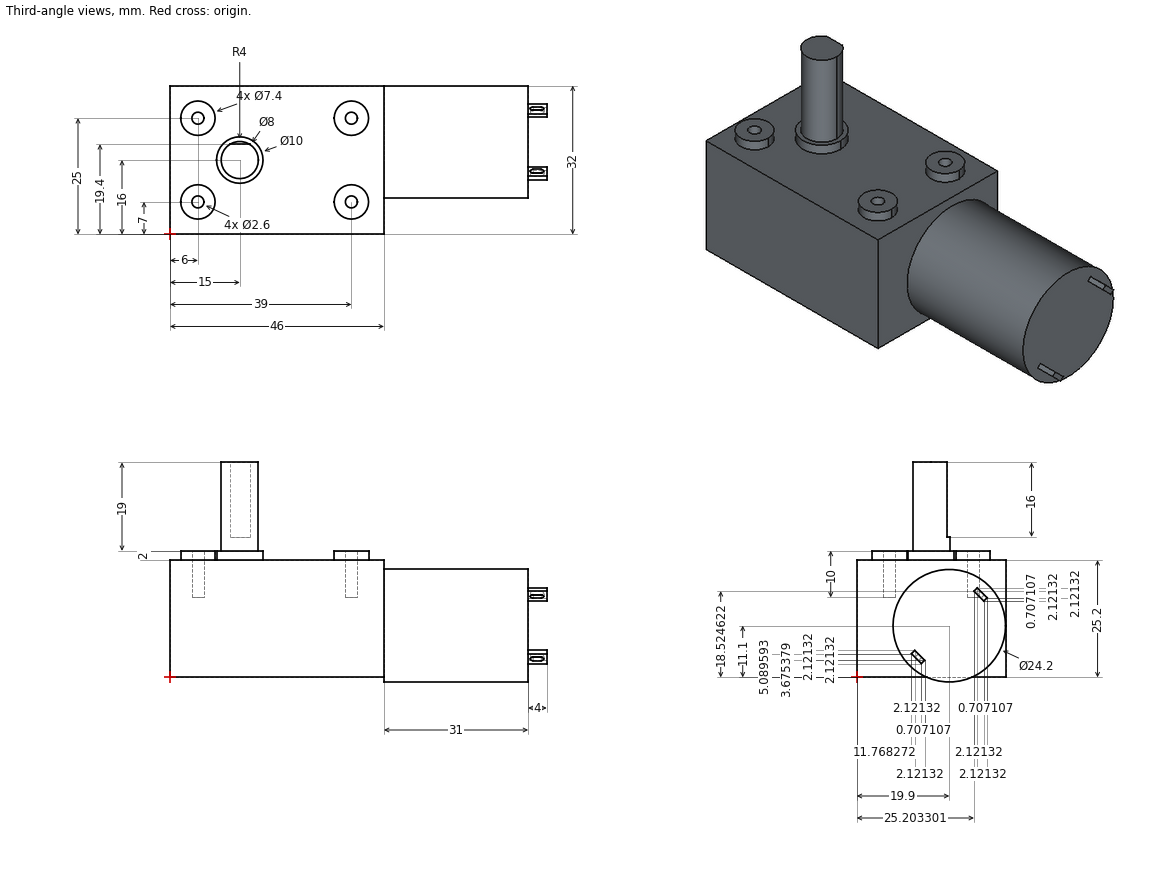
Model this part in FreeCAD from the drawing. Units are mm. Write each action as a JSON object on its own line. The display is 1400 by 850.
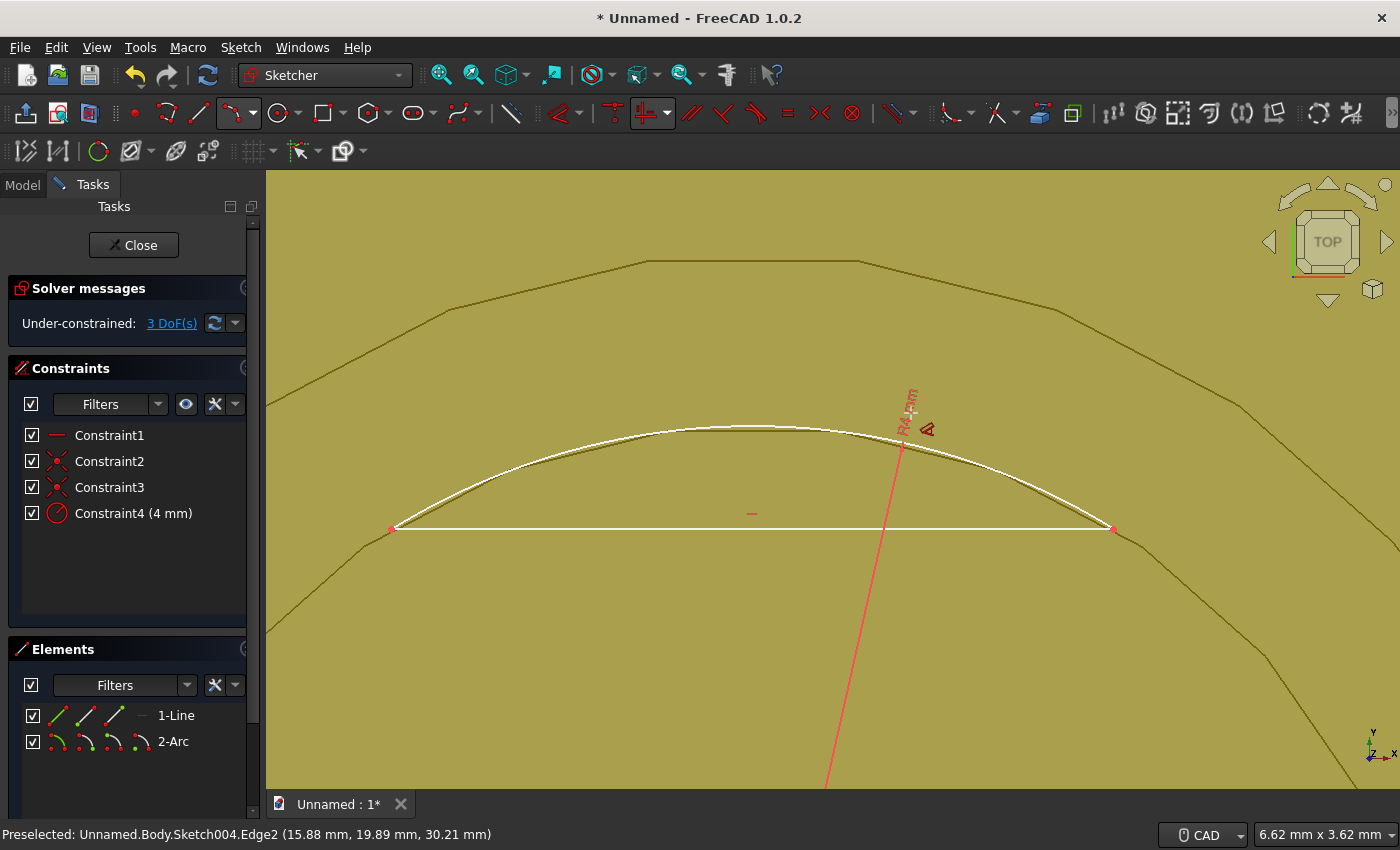
{"action": "scroll", "coordinate": [779, 198], "scroll_direction": "down", "scroll_amount": 3}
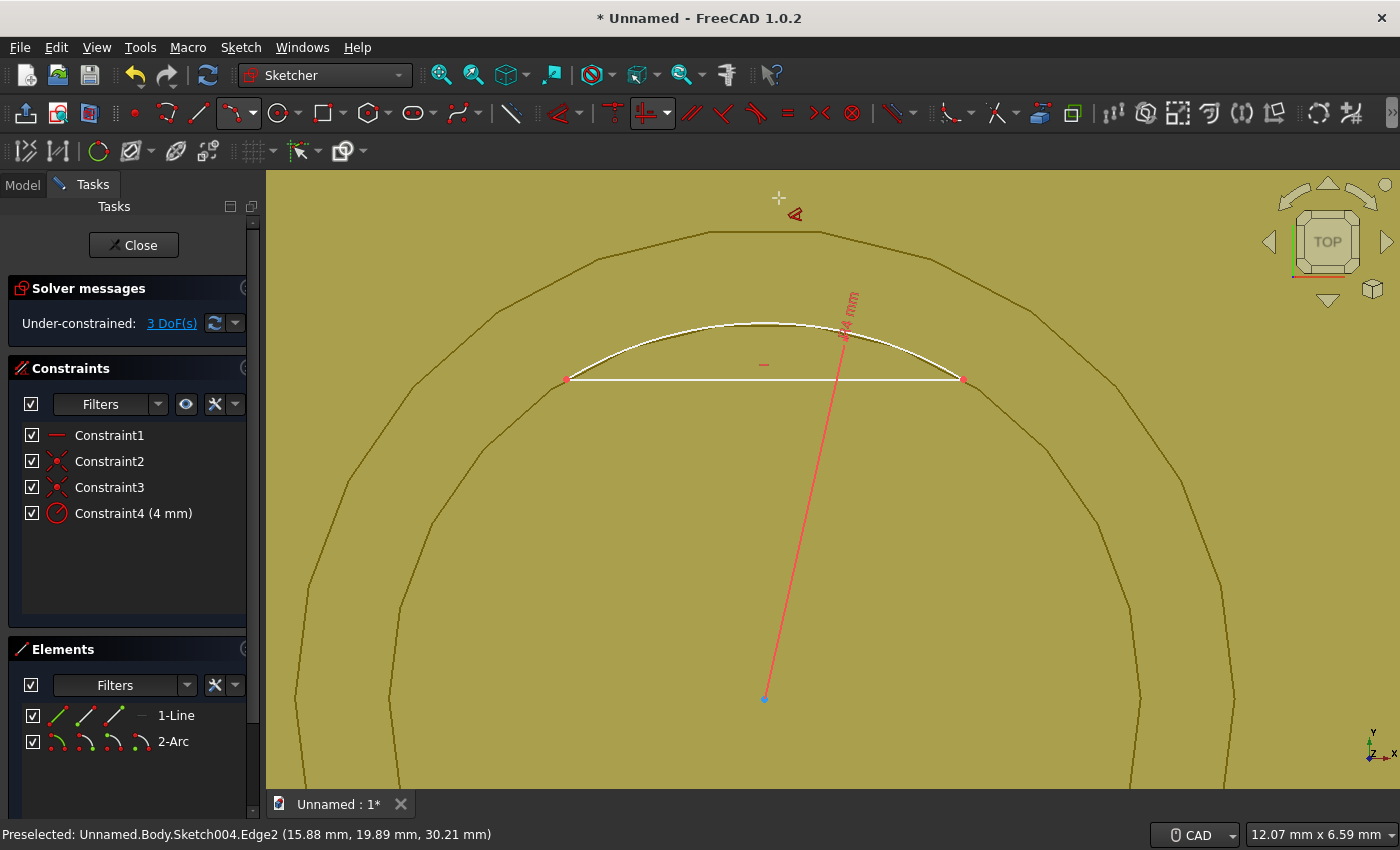
{"action": "left_click", "coordinate": [765, 699]}
{"action": "left_click", "coordinate": [529, 665]}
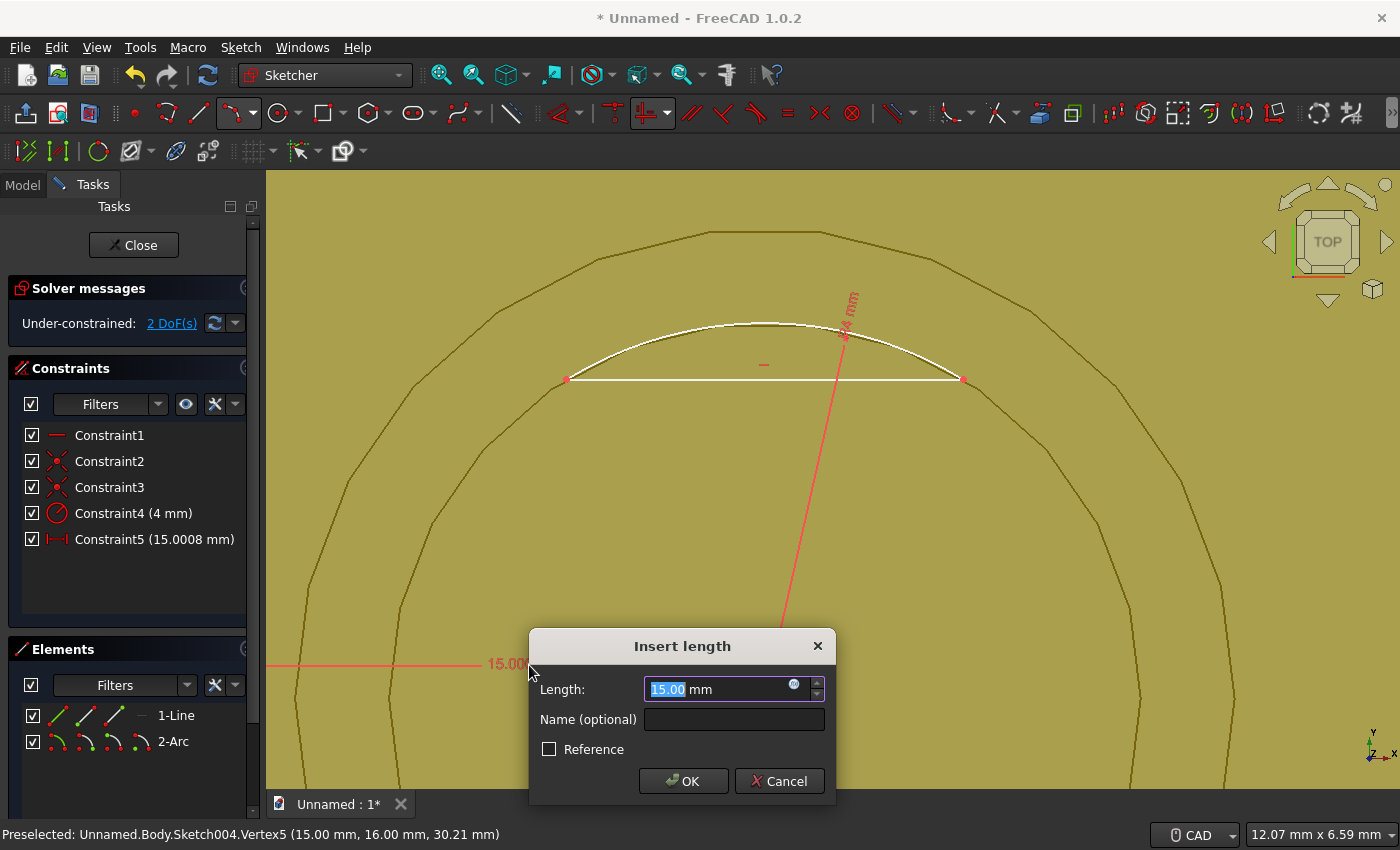
{"action": "type", "text": "15"}
{"action": "key", "text": "Return"}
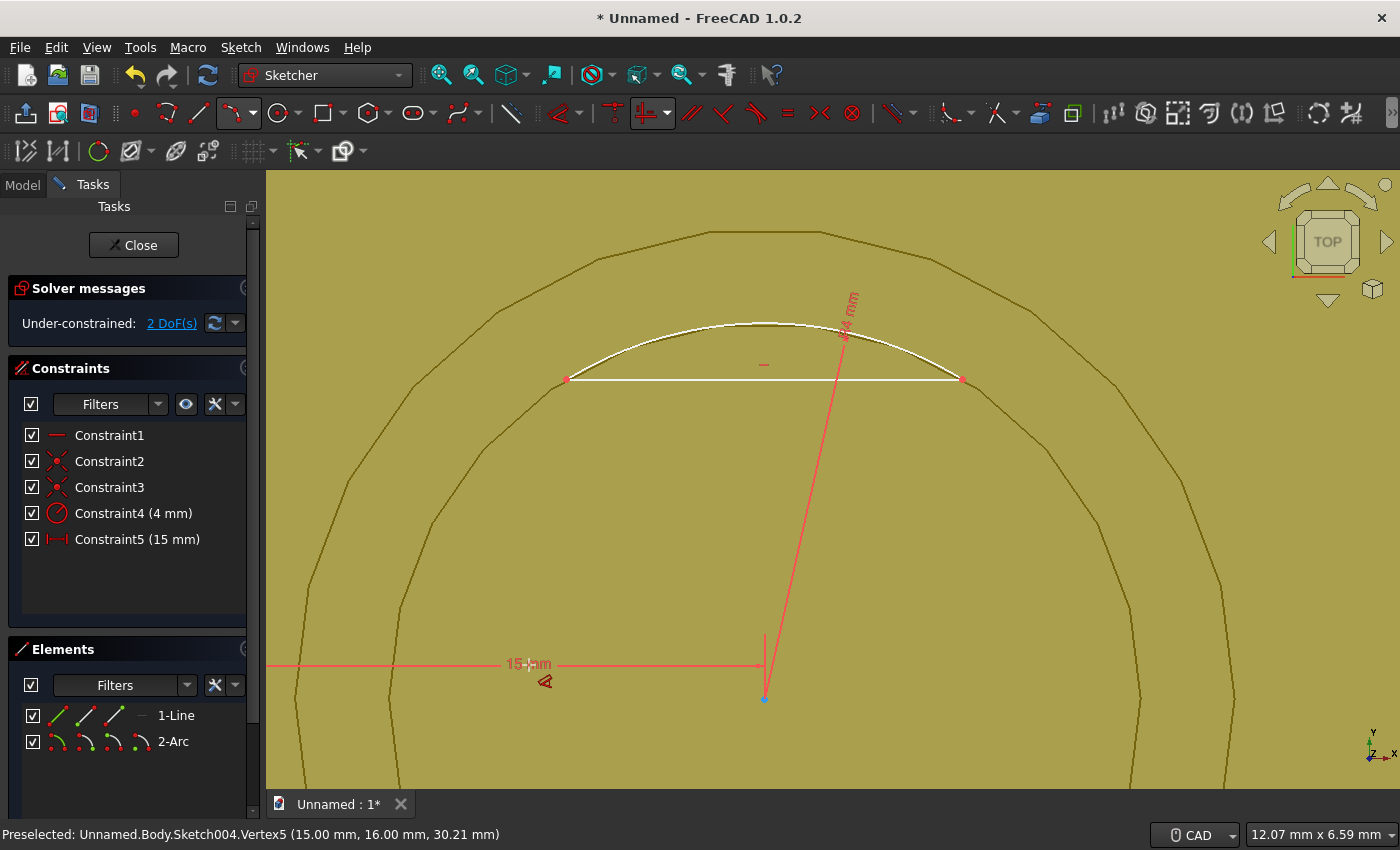
{"action": "left_click", "coordinate": [765, 699]}
{"action": "left_click", "coordinate": [799, 730]}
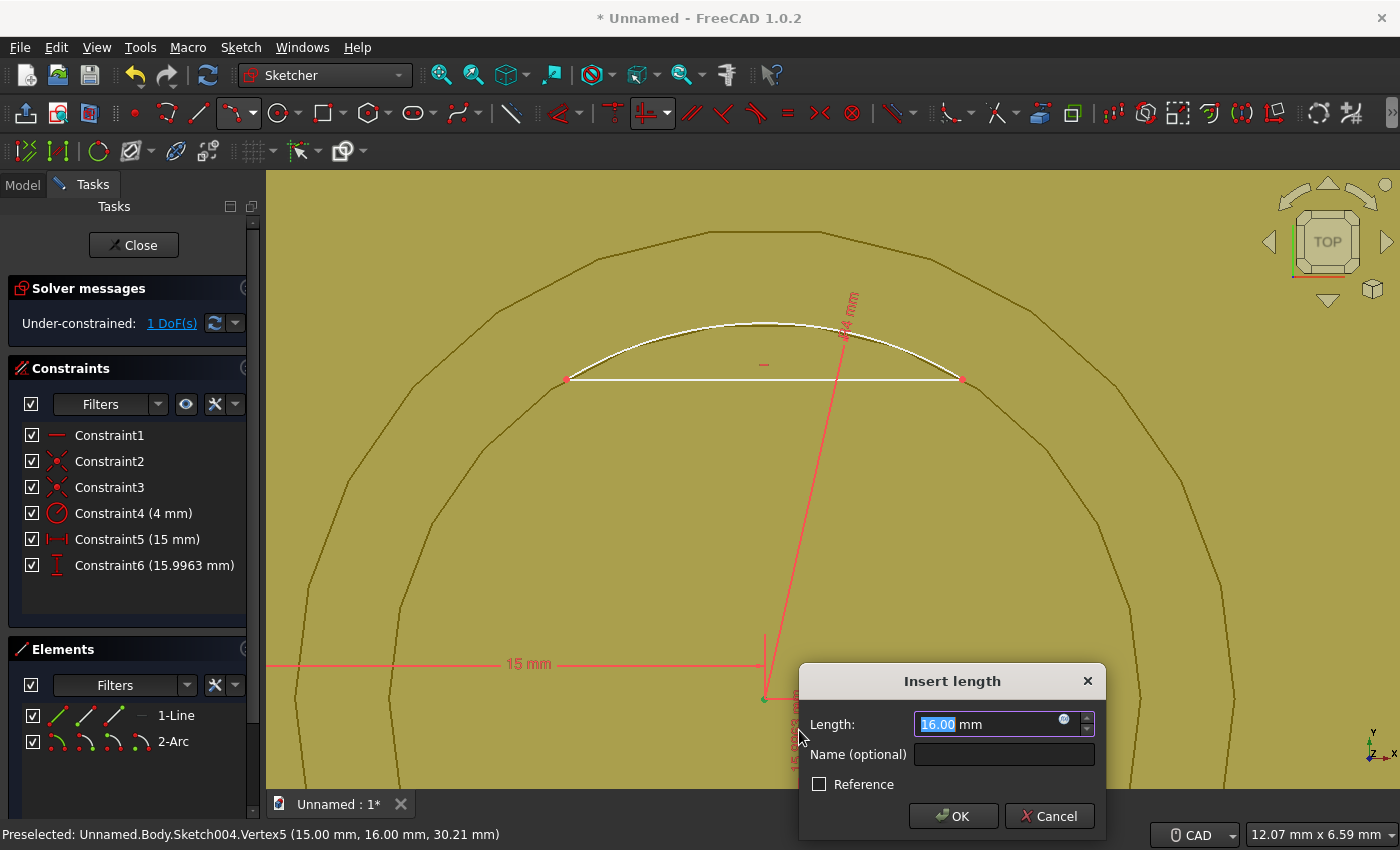
{"action": "type", "text": "16"}
{"action": "key", "text": "Return"}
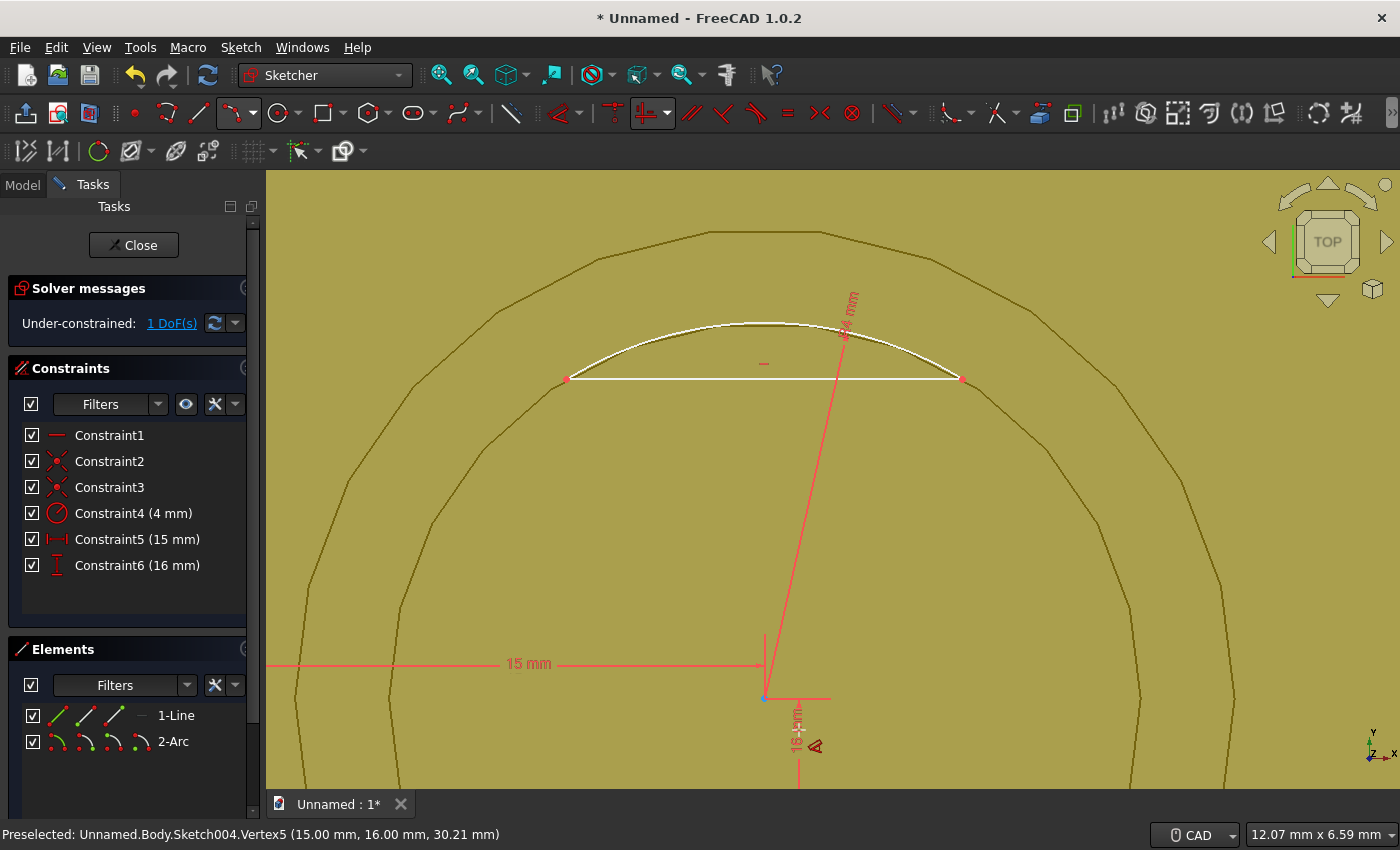
{"action": "left_click", "coordinate": [567, 379]}
{"action": "left_click", "coordinate": [601, 570]}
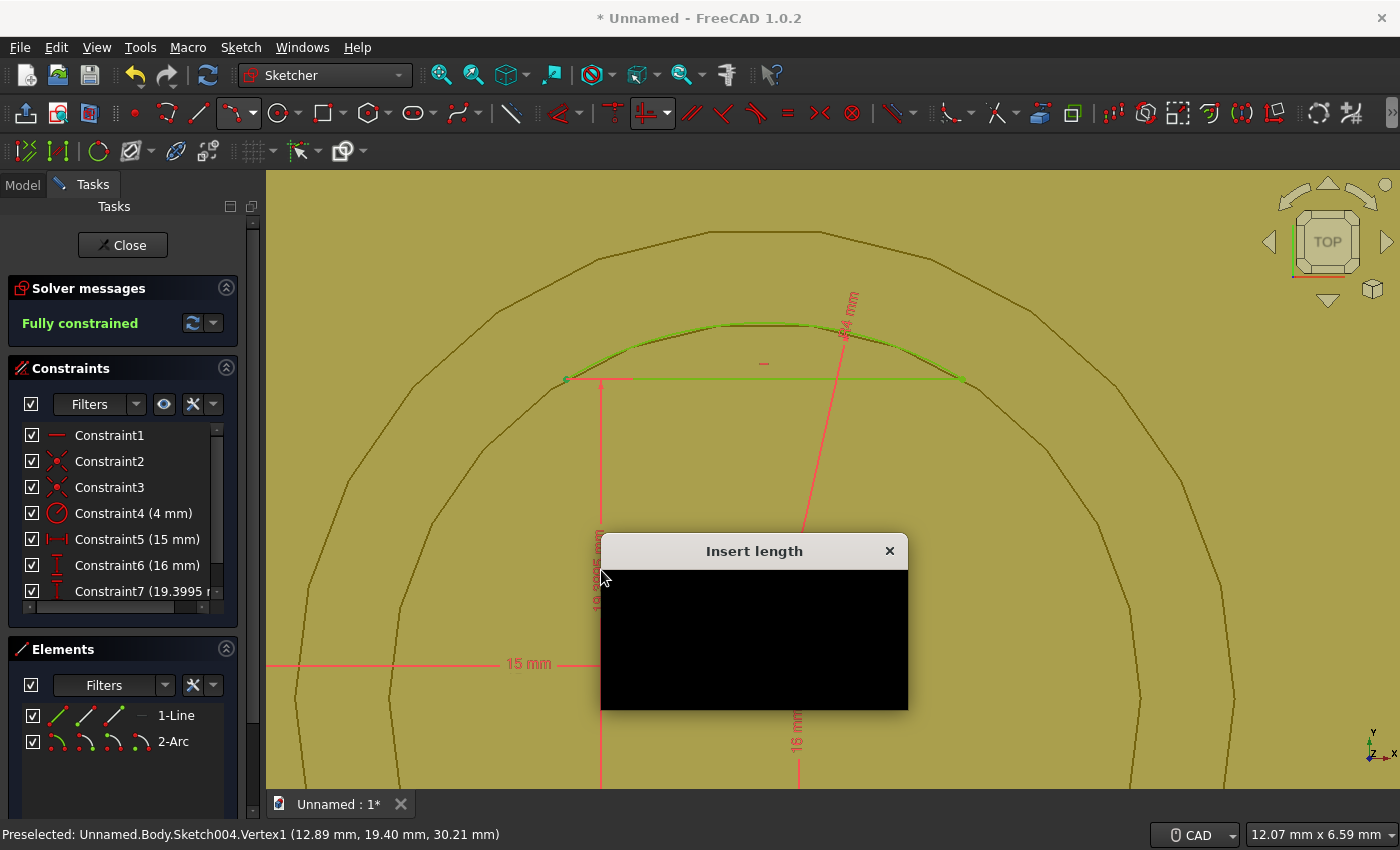
{"action": "type", "text": "19.4"}
{"action": "key", "text": "Return"}
{"action": "key", "text": "Escape"}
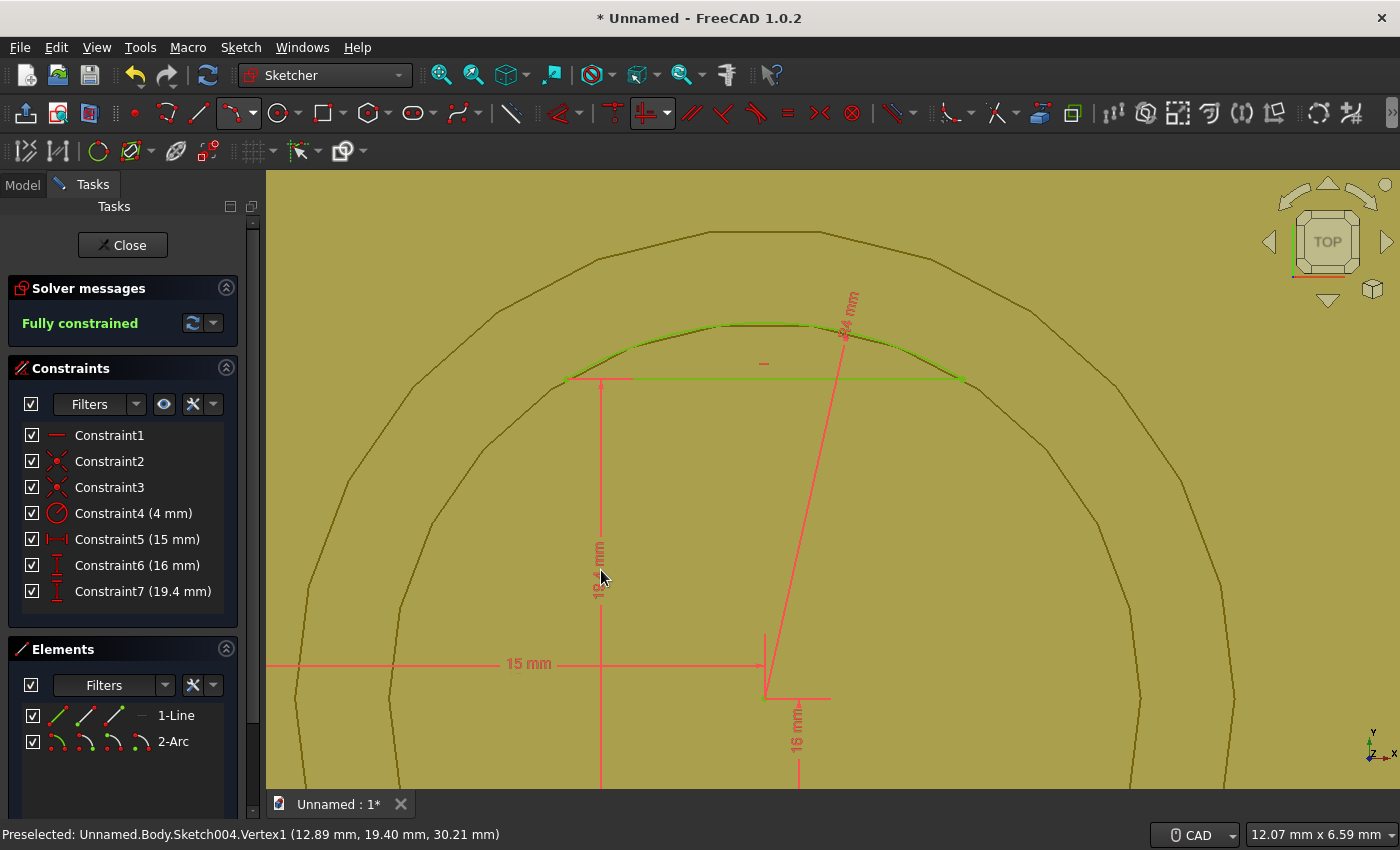
{"action": "left_click", "coordinate": [123, 245]}